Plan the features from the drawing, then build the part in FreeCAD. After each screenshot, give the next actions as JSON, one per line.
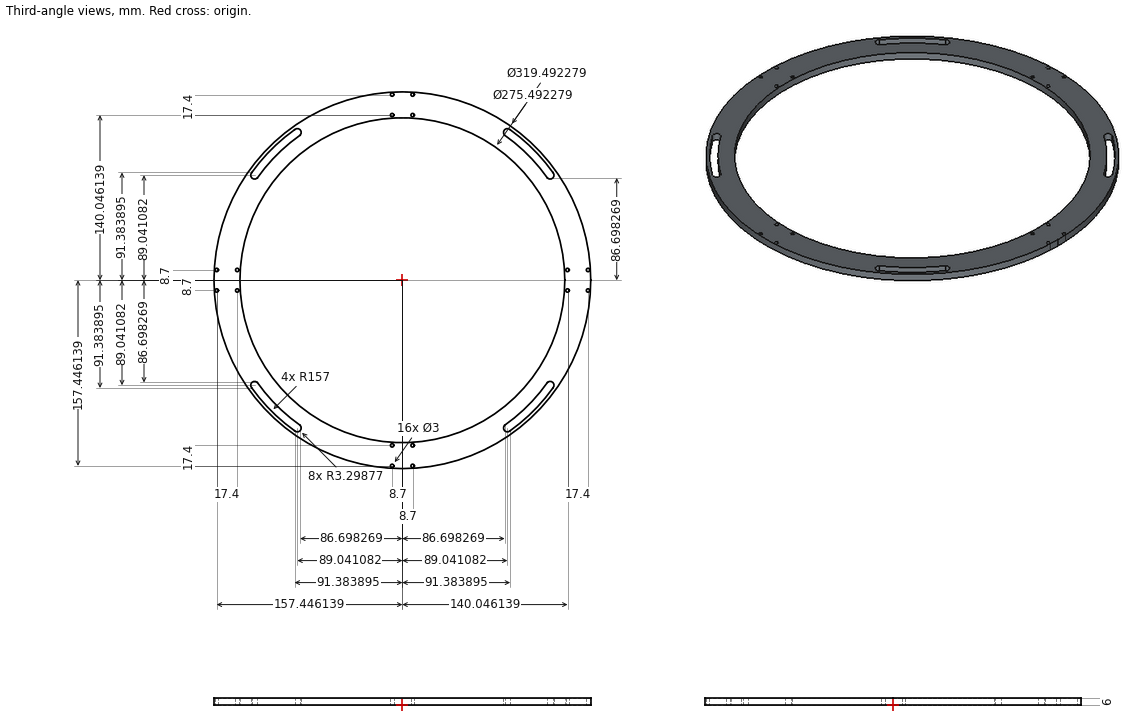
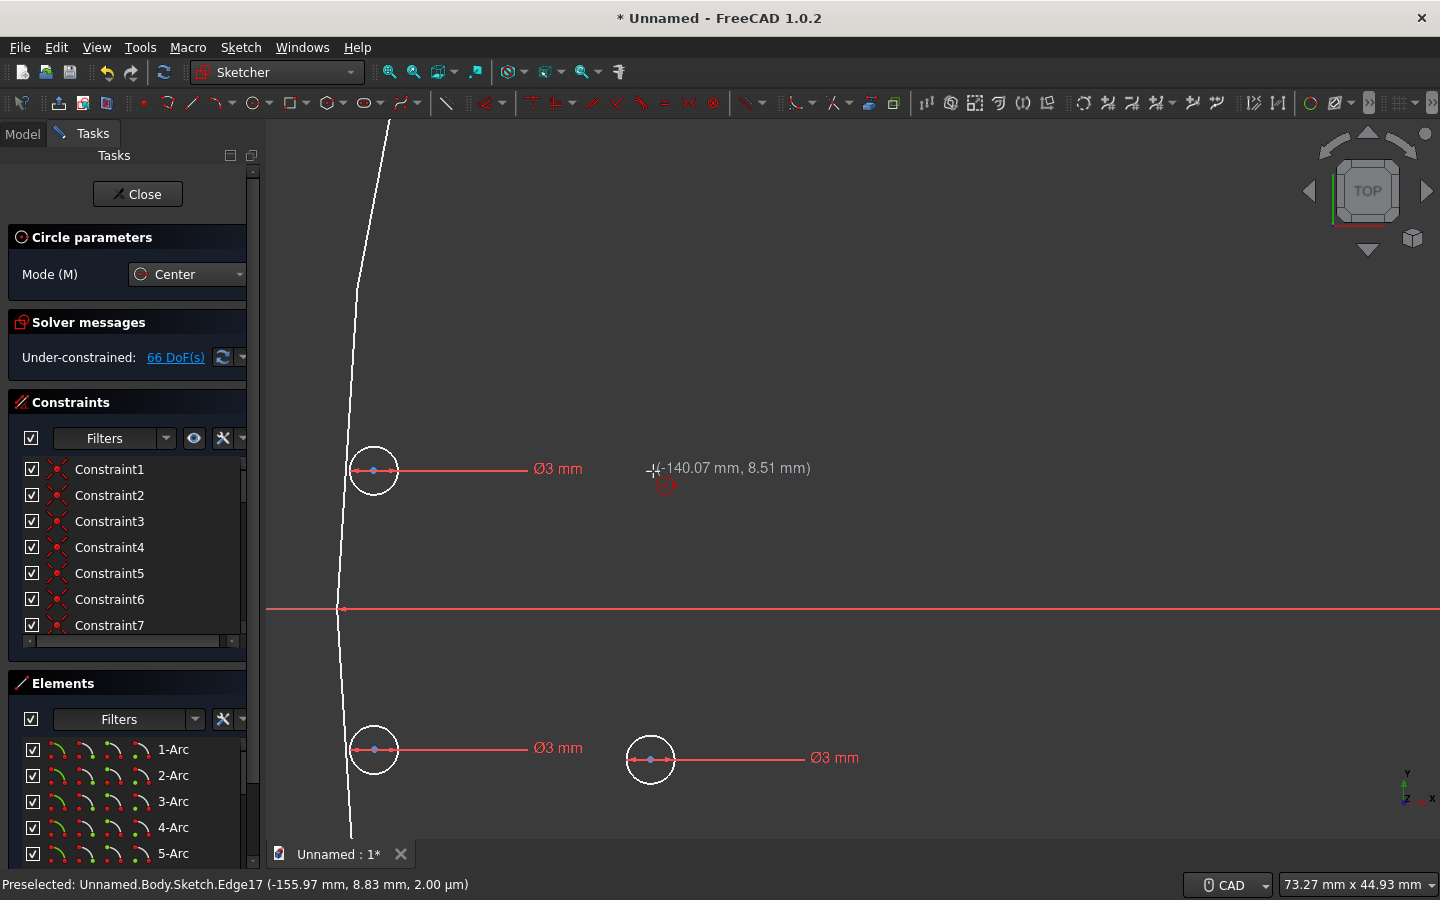
{"action": "scroll", "coordinate": [574, 466], "scroll_direction": "down", "scroll_amount": 12}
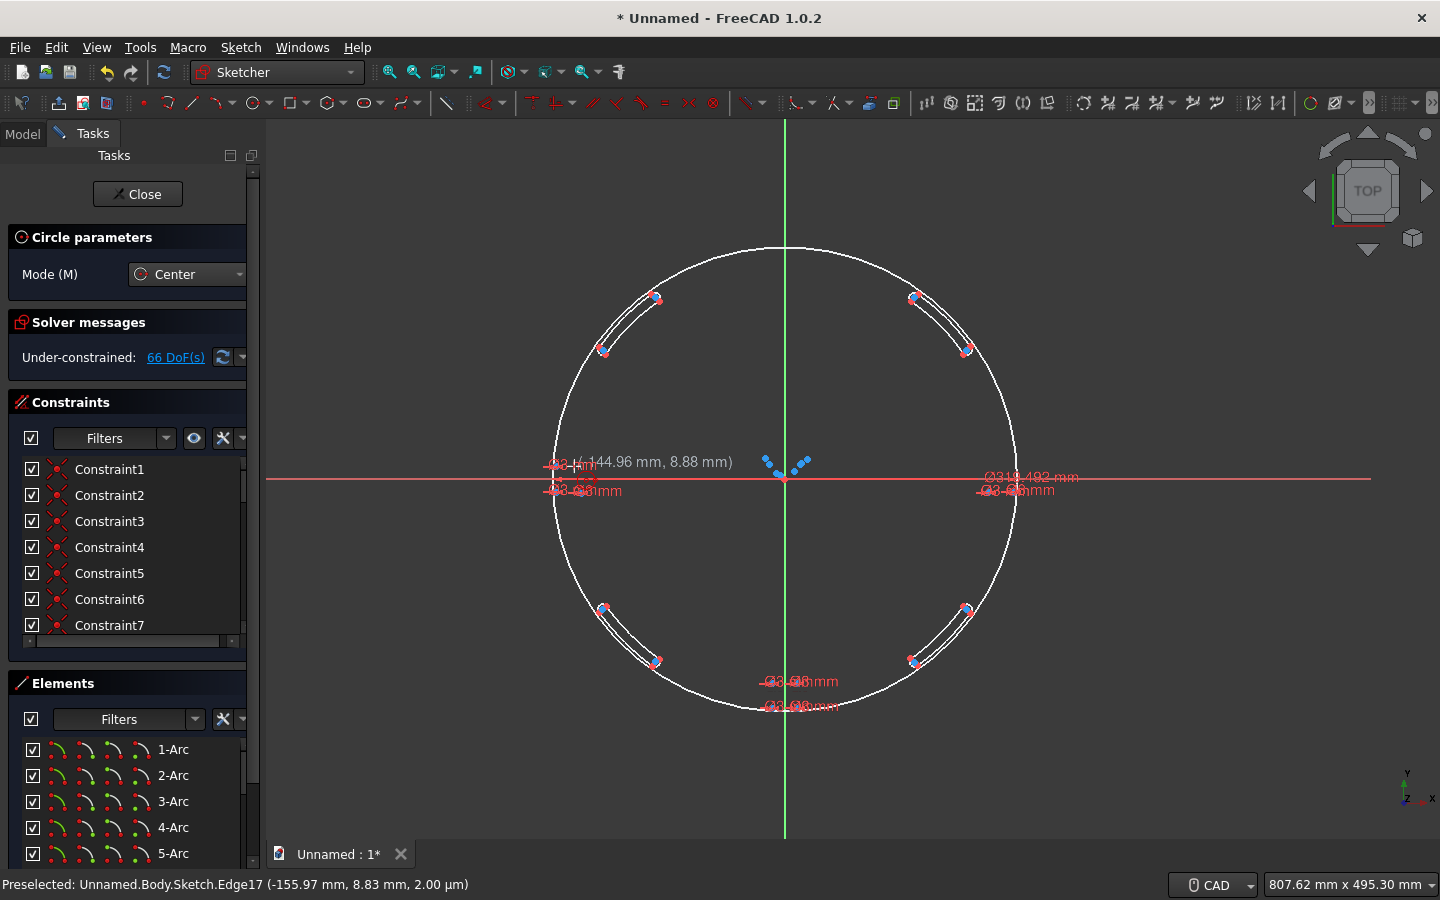
{"action": "scroll", "coordinate": [581, 467], "scroll_direction": "up", "scroll_amount": 2}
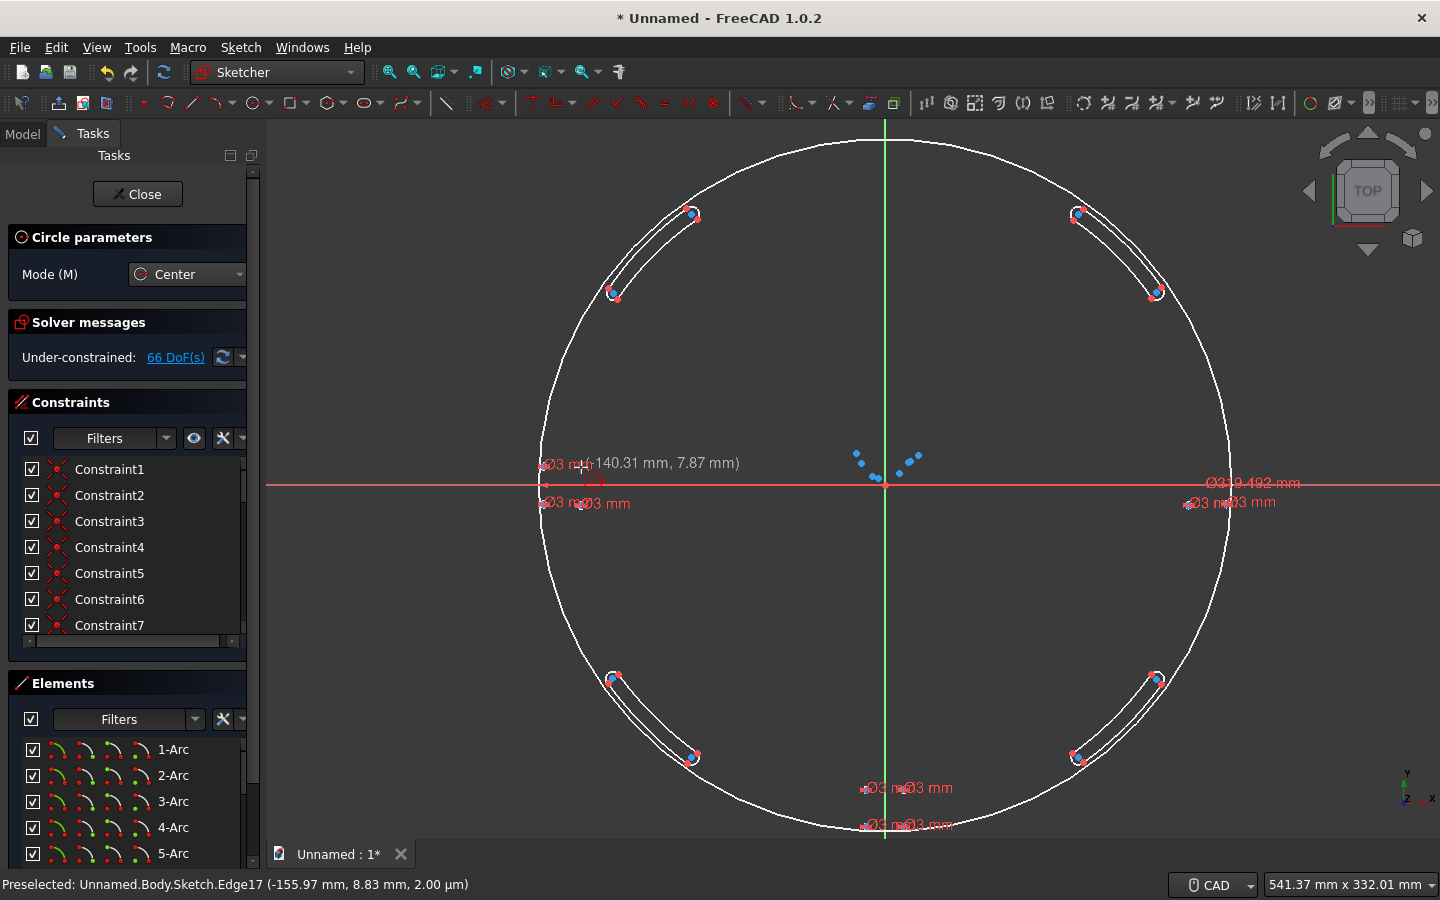
{"action": "left_click", "coordinate": [581, 466]}
{"action": "mouse_move", "coordinate": [584, 464]}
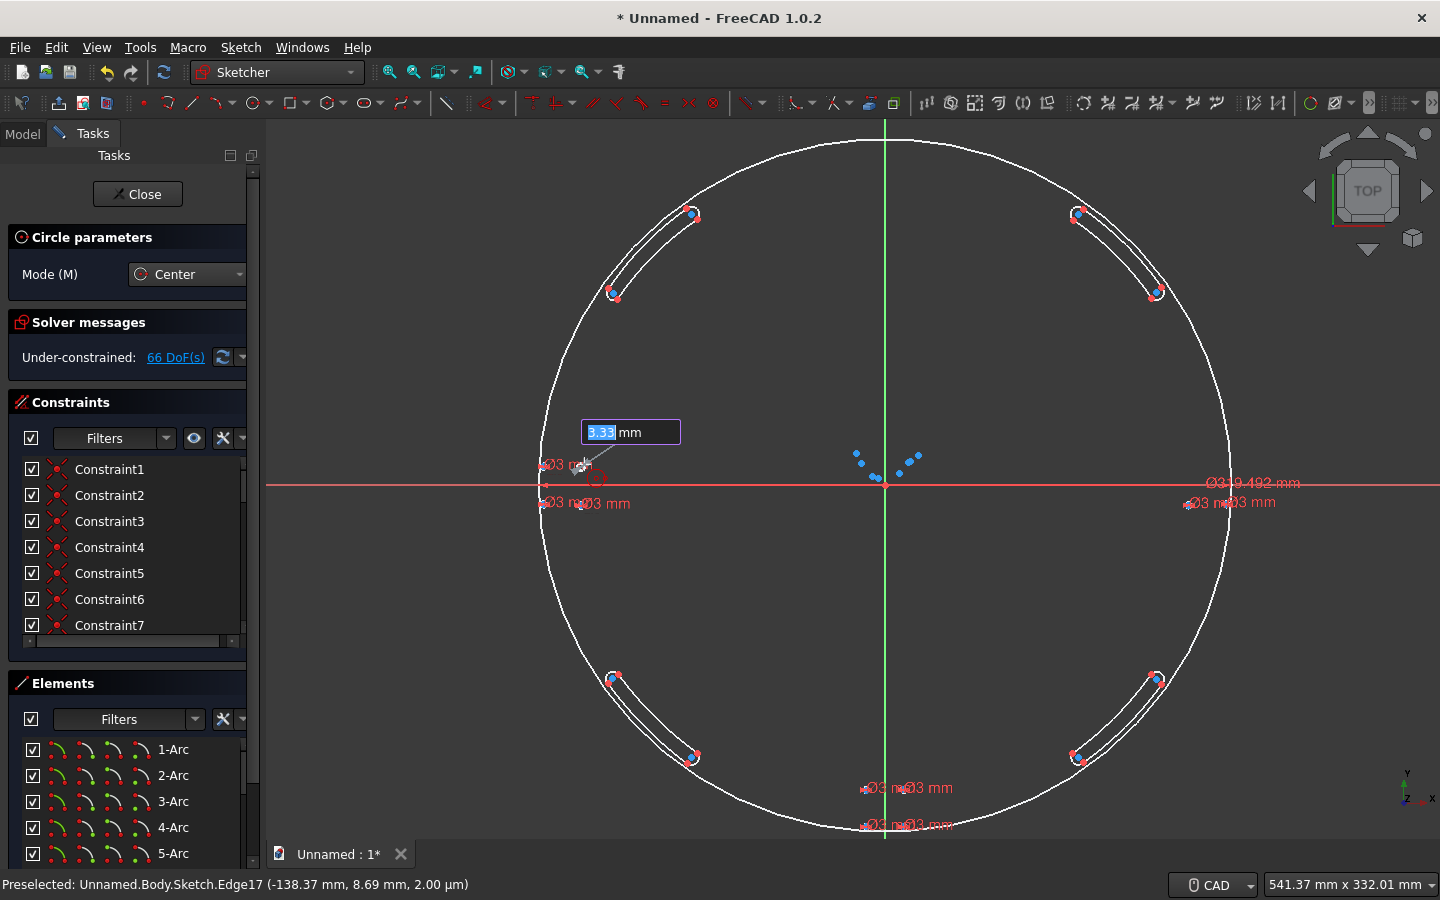
{"action": "type", "text": "3"}
{"action": "key", "text": "Return"}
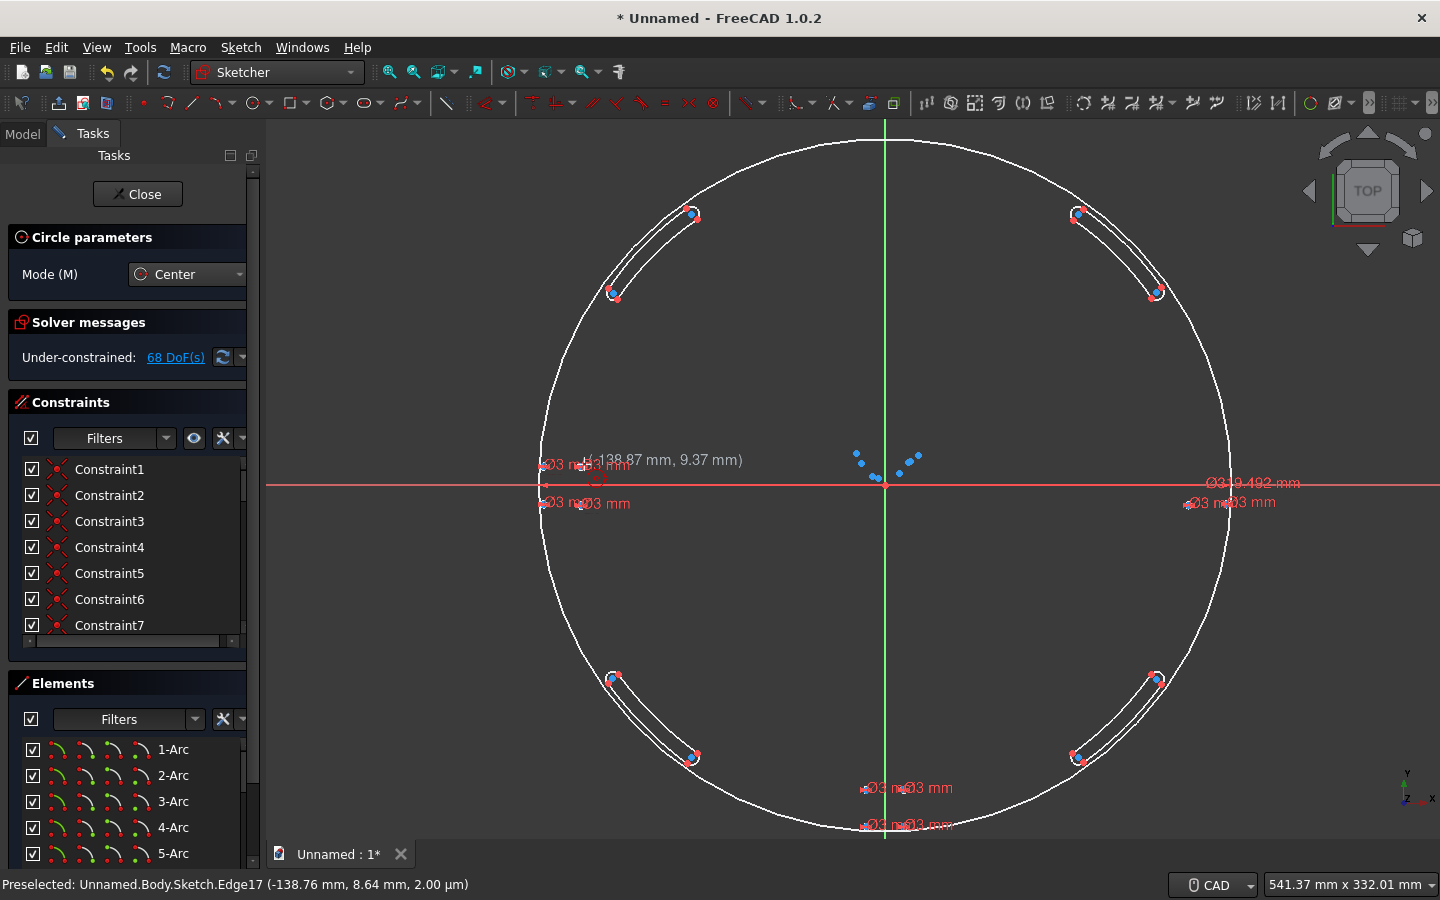
{"action": "scroll", "coordinate": [866, 182], "scroll_direction": "up", "scroll_amount": 10}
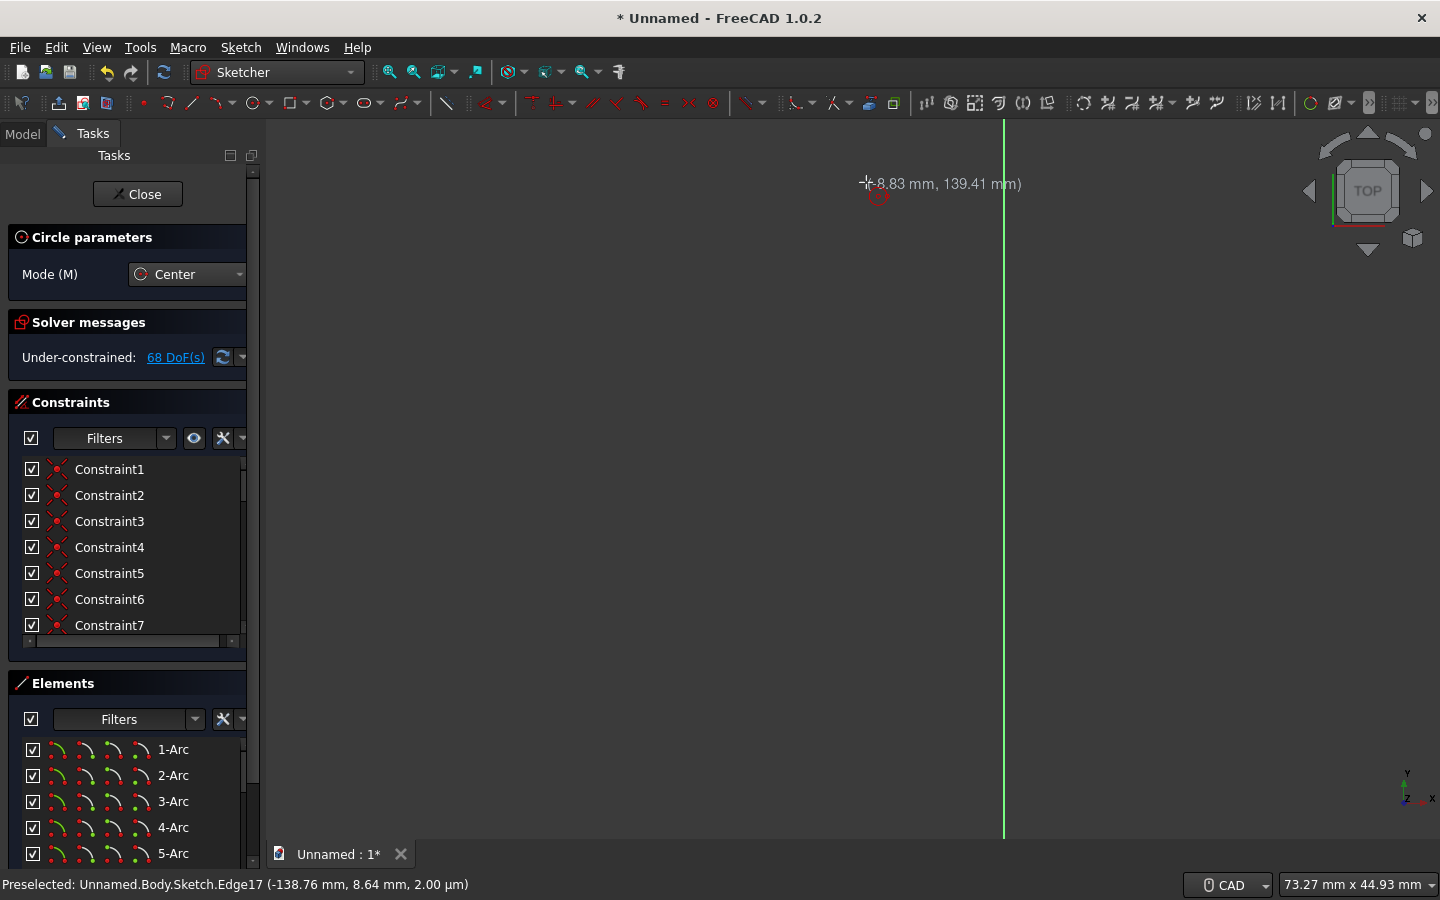
{"action": "scroll", "coordinate": [763, 285], "scroll_direction": "down", "scroll_amount": 12}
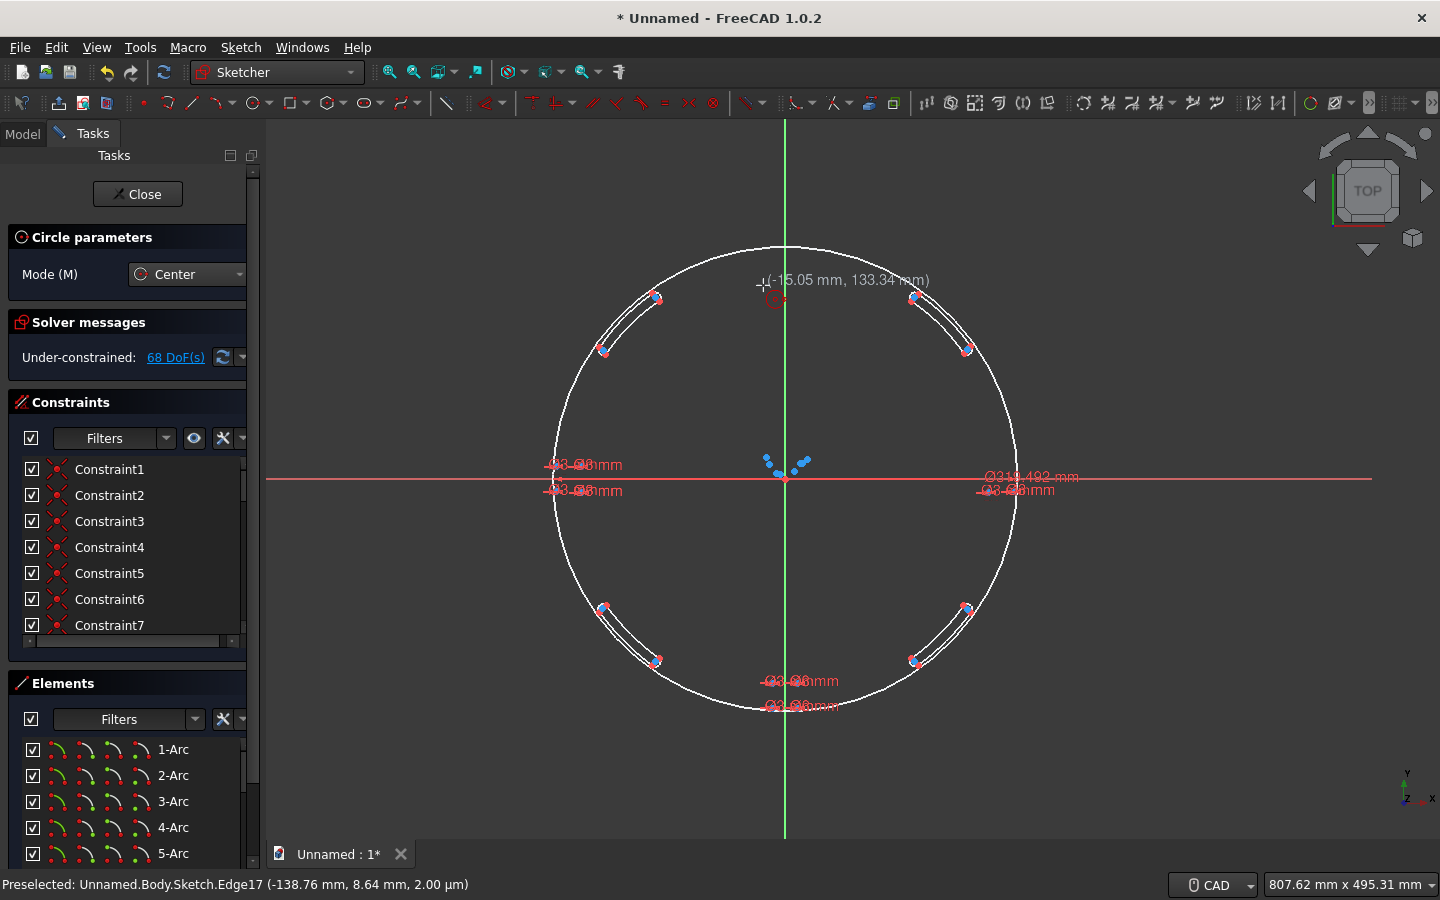
{"action": "scroll", "coordinate": [773, 276], "scroll_direction": "up", "scroll_amount": 2}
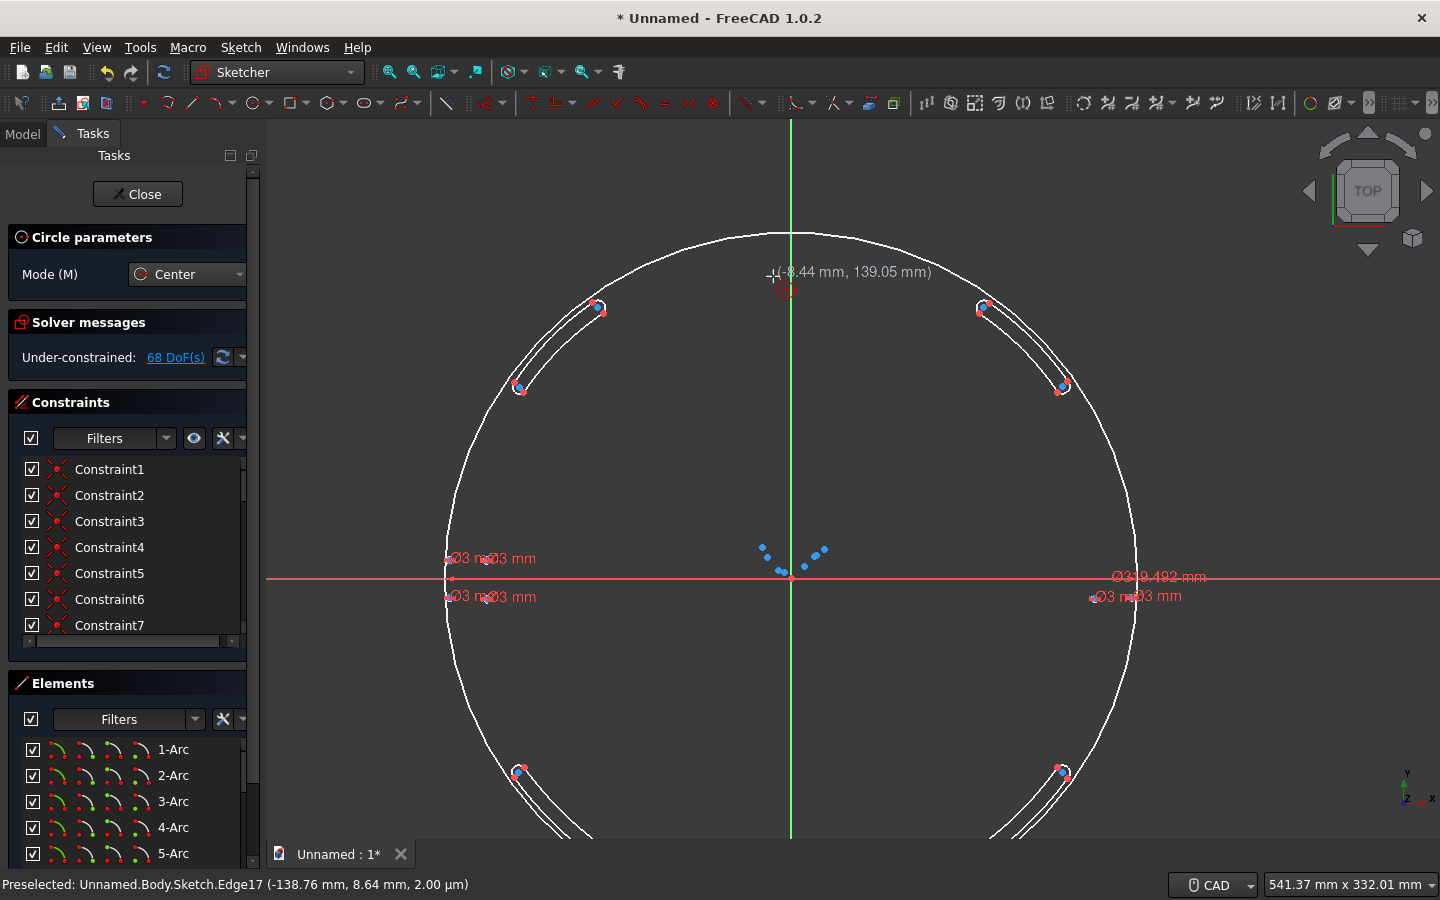
{"action": "left_click", "coordinate": [772, 275]}
{"action": "mouse_move", "coordinate": [775, 273]}